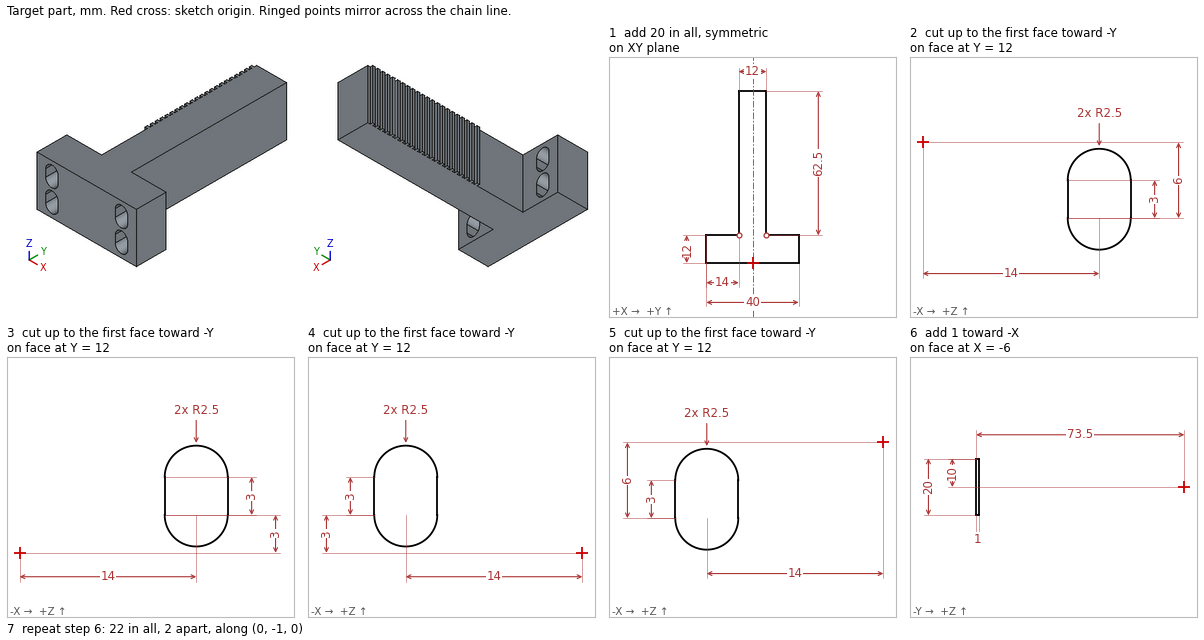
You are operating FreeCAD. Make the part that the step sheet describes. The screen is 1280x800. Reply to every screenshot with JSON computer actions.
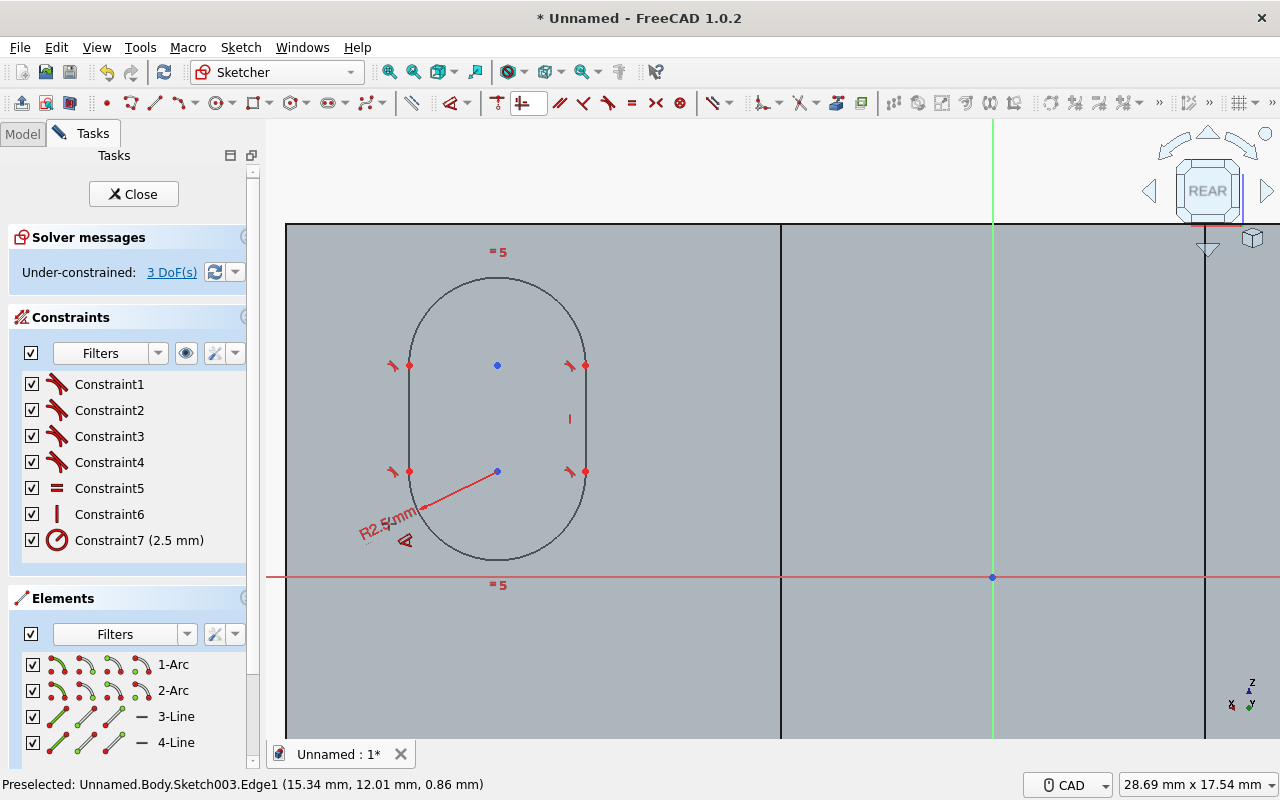
{"action": "left_click", "coordinate": [409, 440]}
{"action": "left_click", "coordinate": [375, 419]}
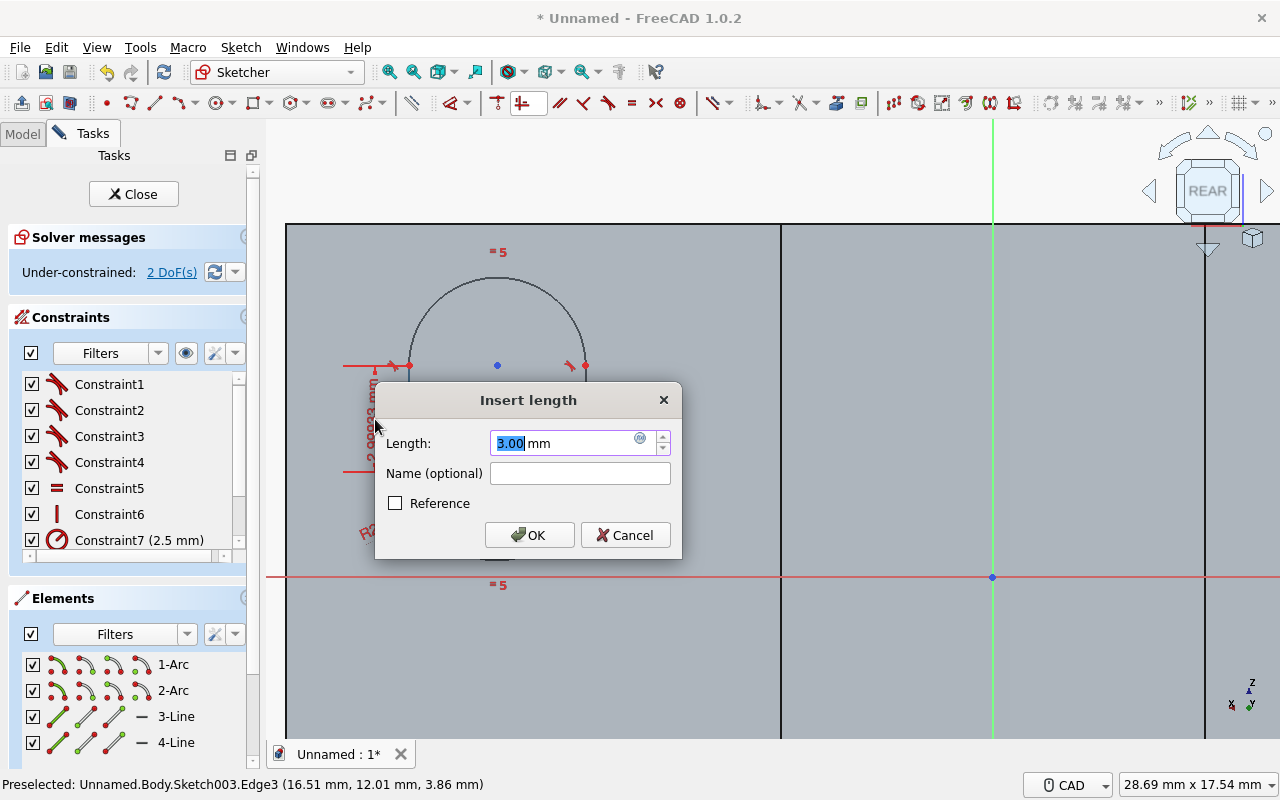
{"action": "type", "text": "3"}
{"action": "key", "text": "Return"}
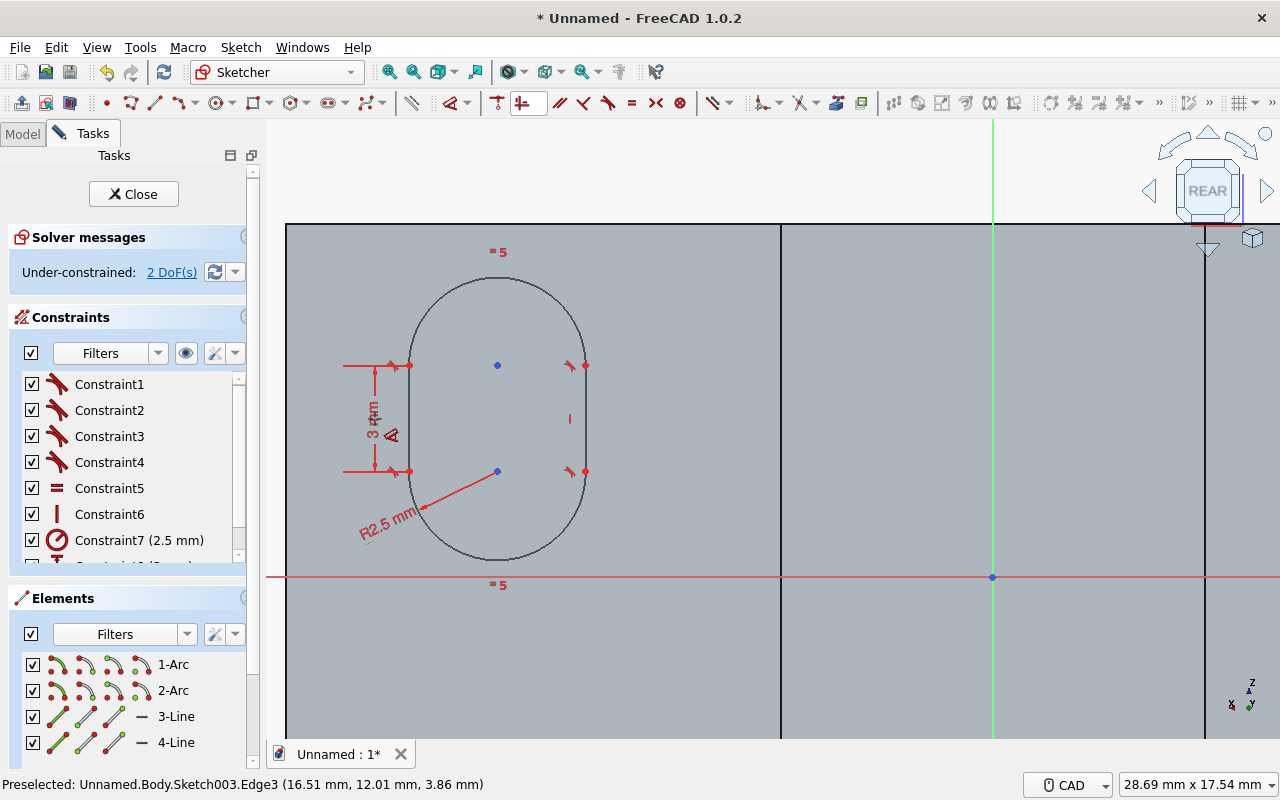
{"action": "left_click", "coordinate": [409, 472]}
{"action": "left_click", "coordinate": [375, 500]}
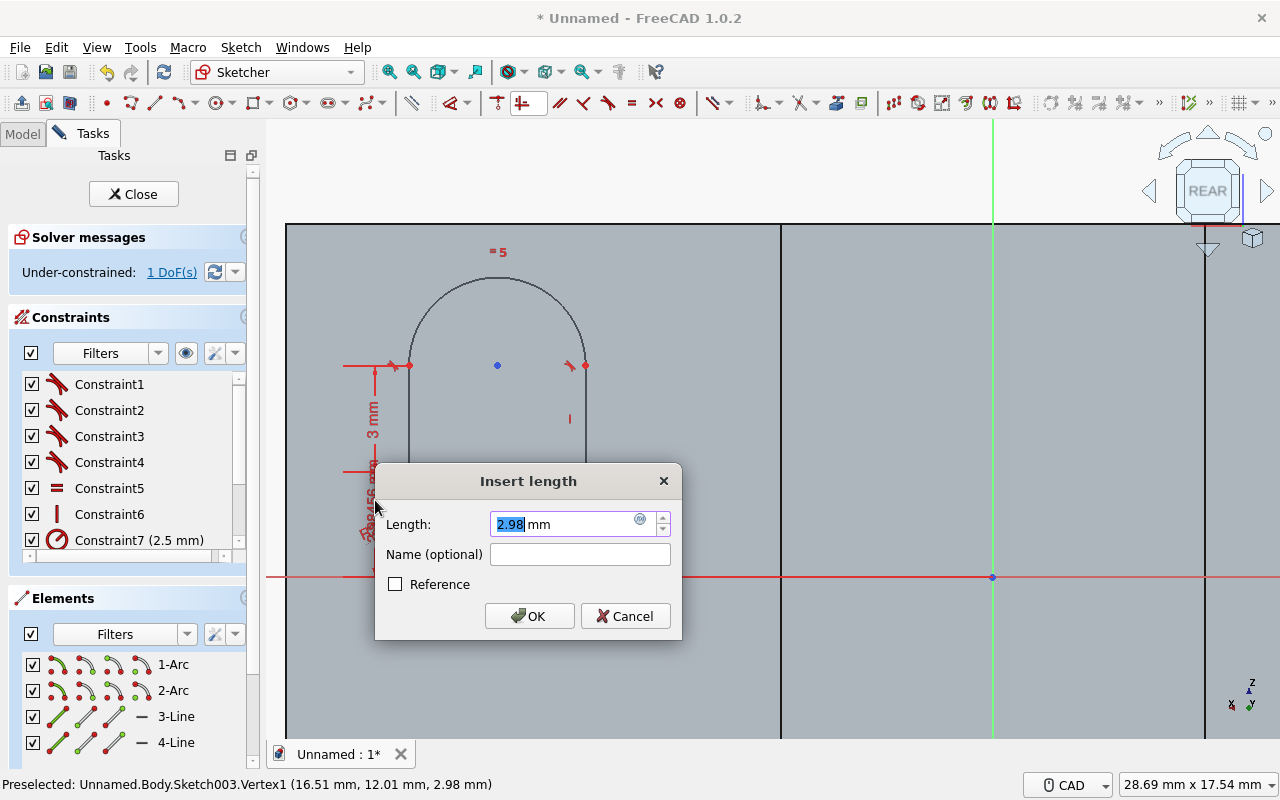
{"action": "type", "text": "3"}
{"action": "key", "text": "Return"}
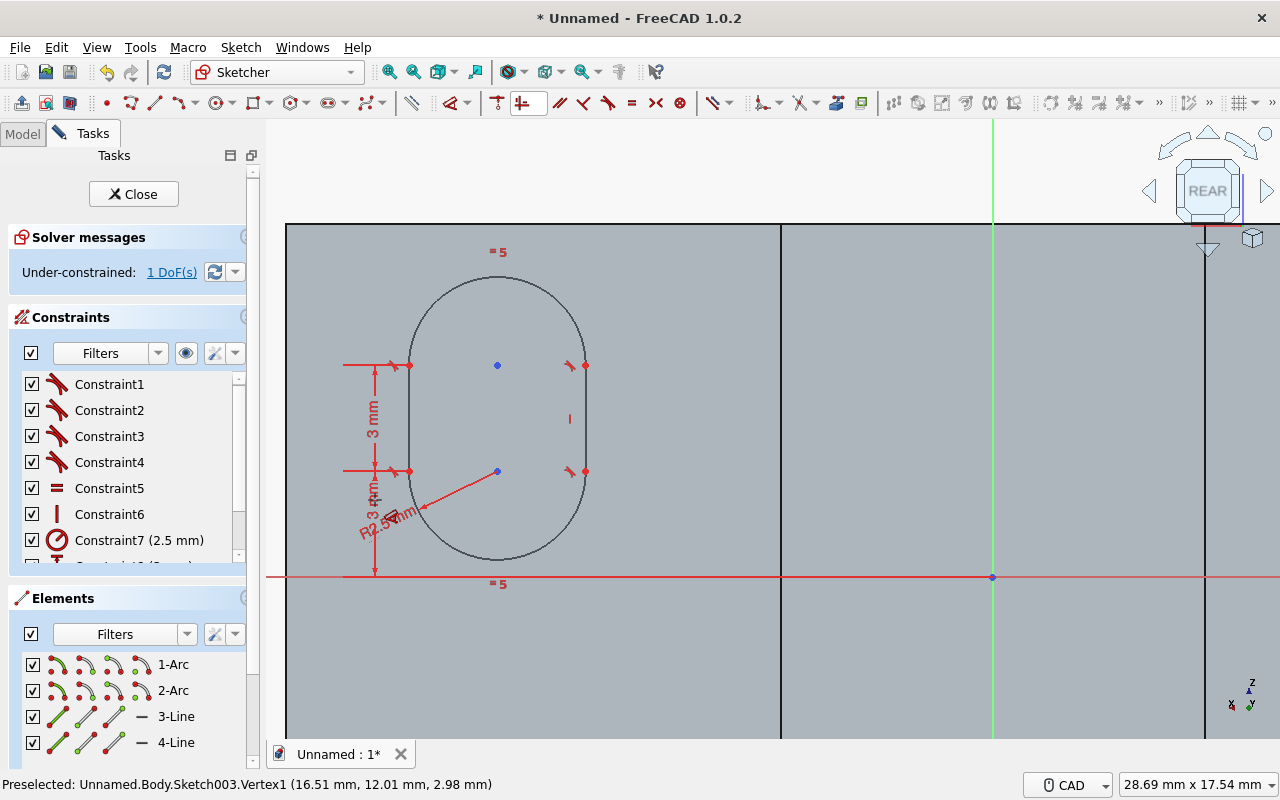
{"action": "left_click", "coordinate": [497, 471]}
{"action": "left_click", "coordinate": [745, 611]}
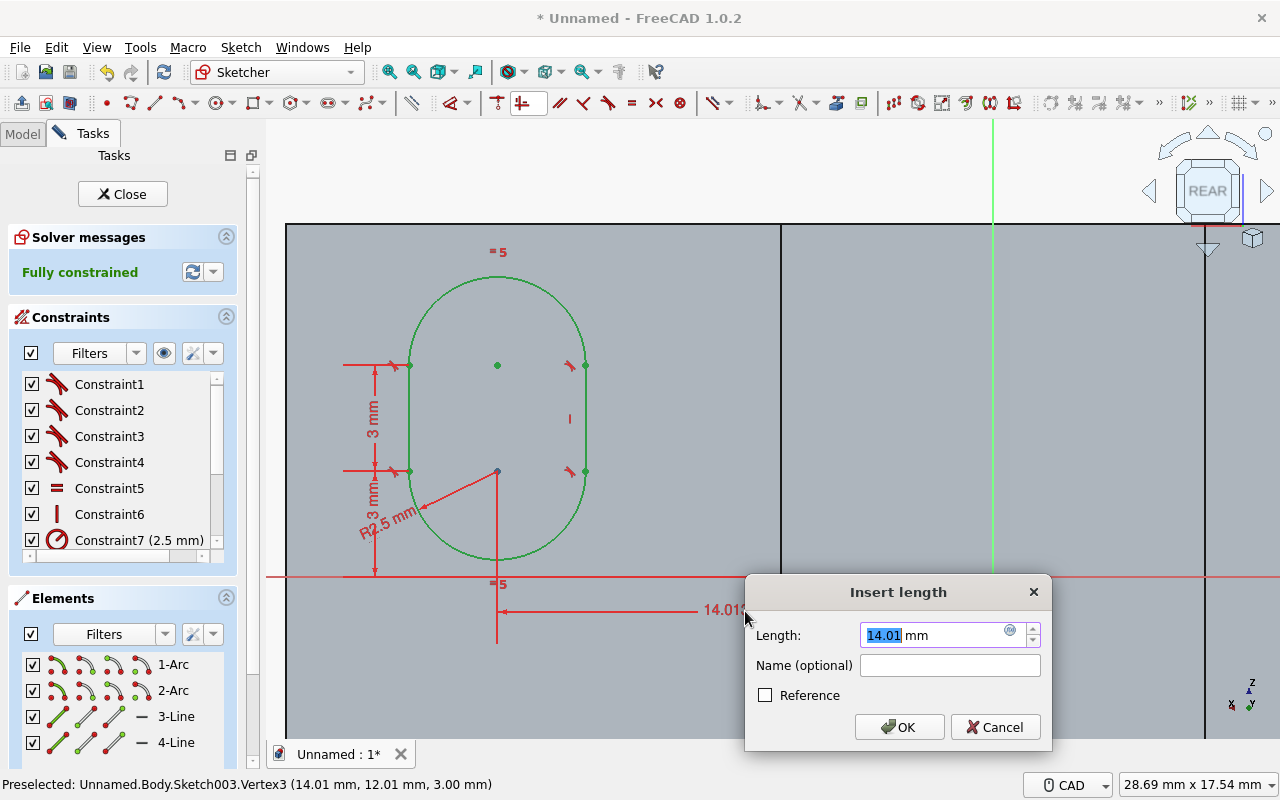
{"action": "type", "text": "14"}
{"action": "key", "text": "Return"}
{"action": "key", "text": "Escape"}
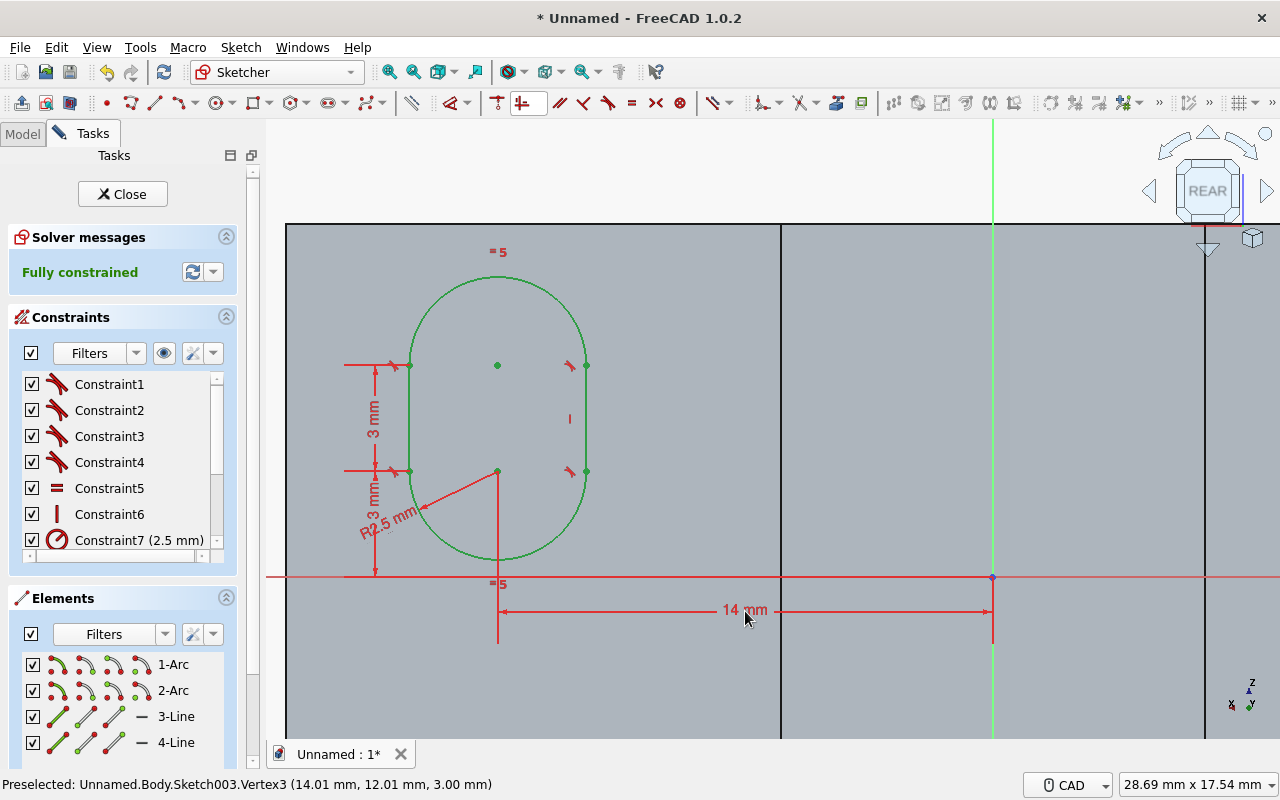
{"action": "left_click", "coordinate": [123, 194]}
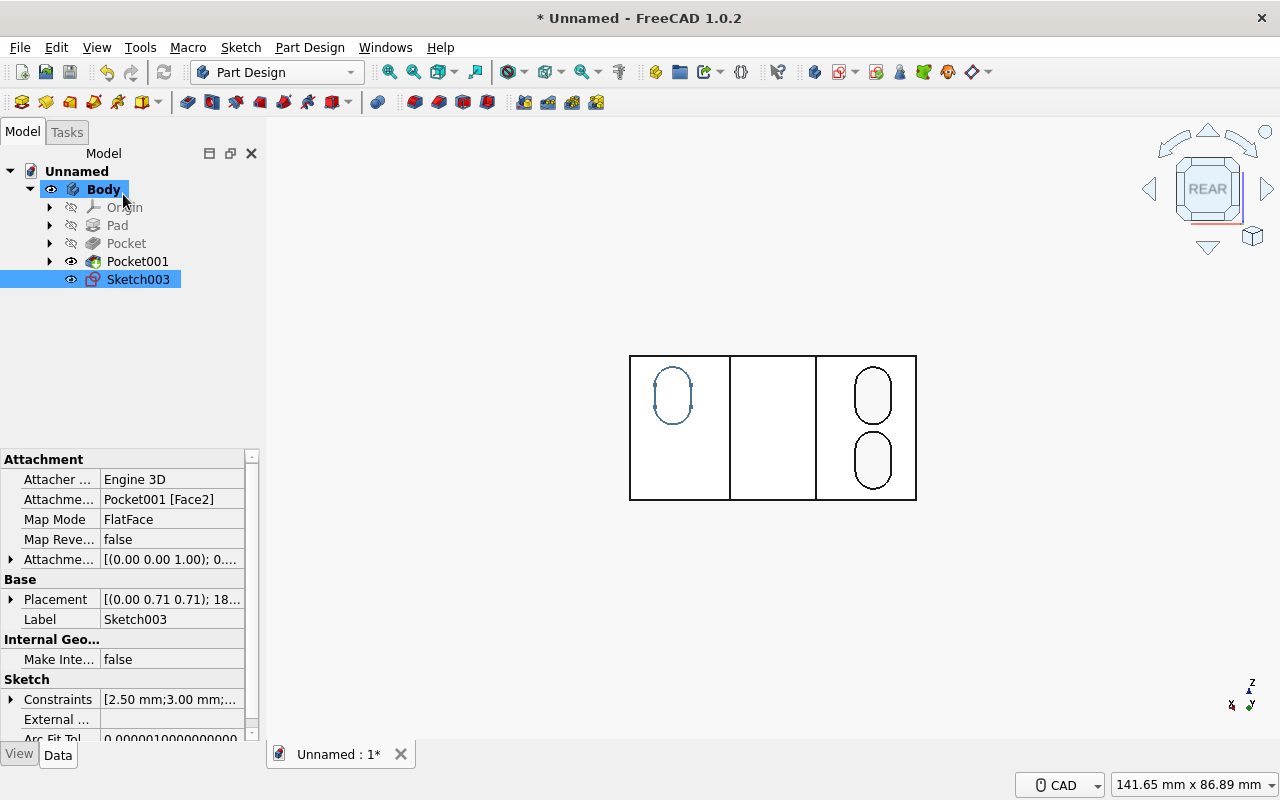
{"action": "left_click", "coordinate": [188, 102]}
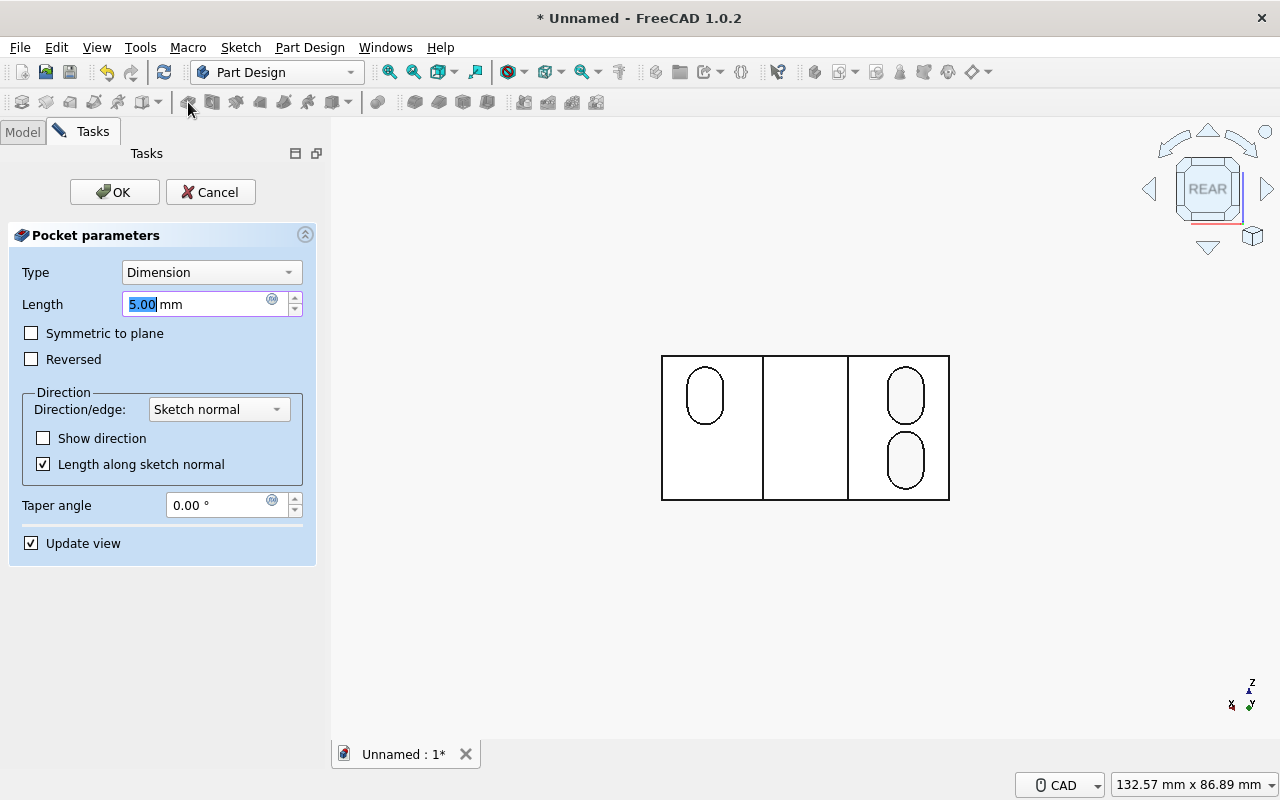
{"action": "left_click", "coordinate": [212, 272]}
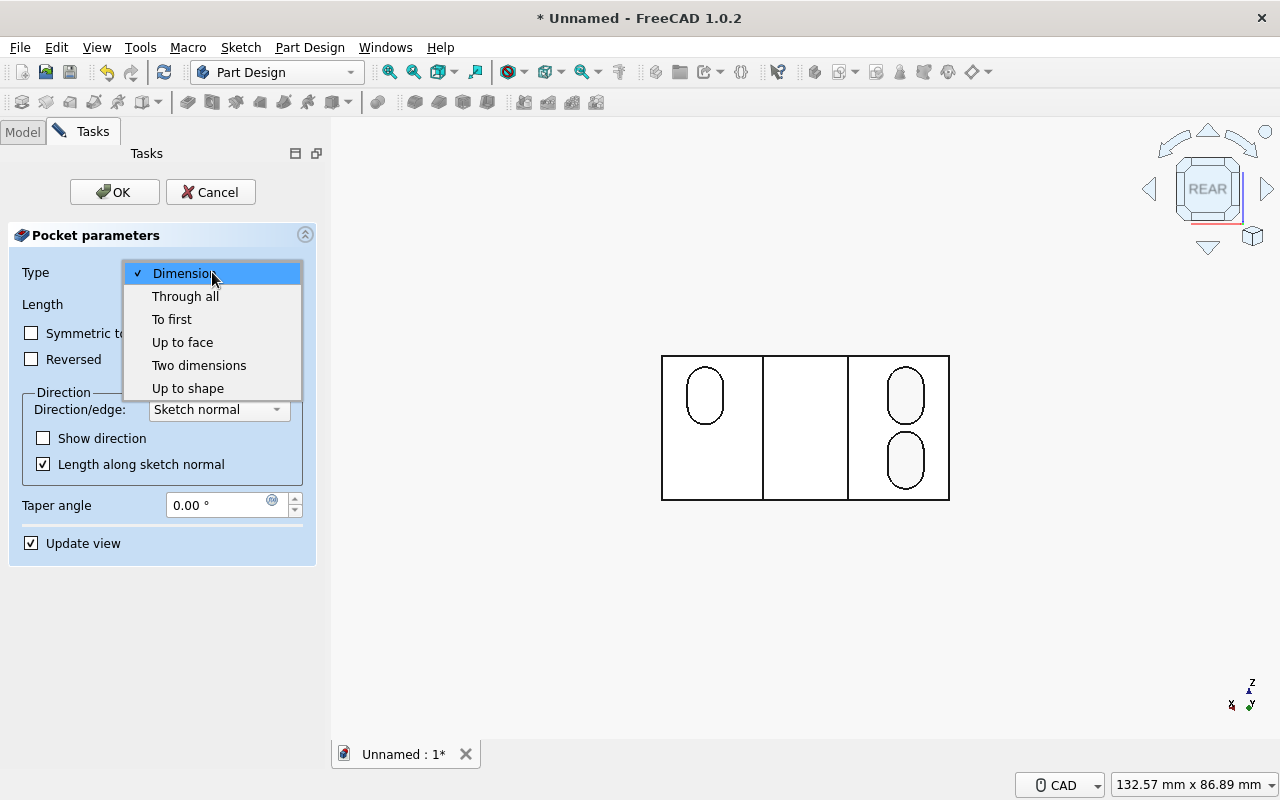
{"action": "left_click", "coordinate": [212, 320]}